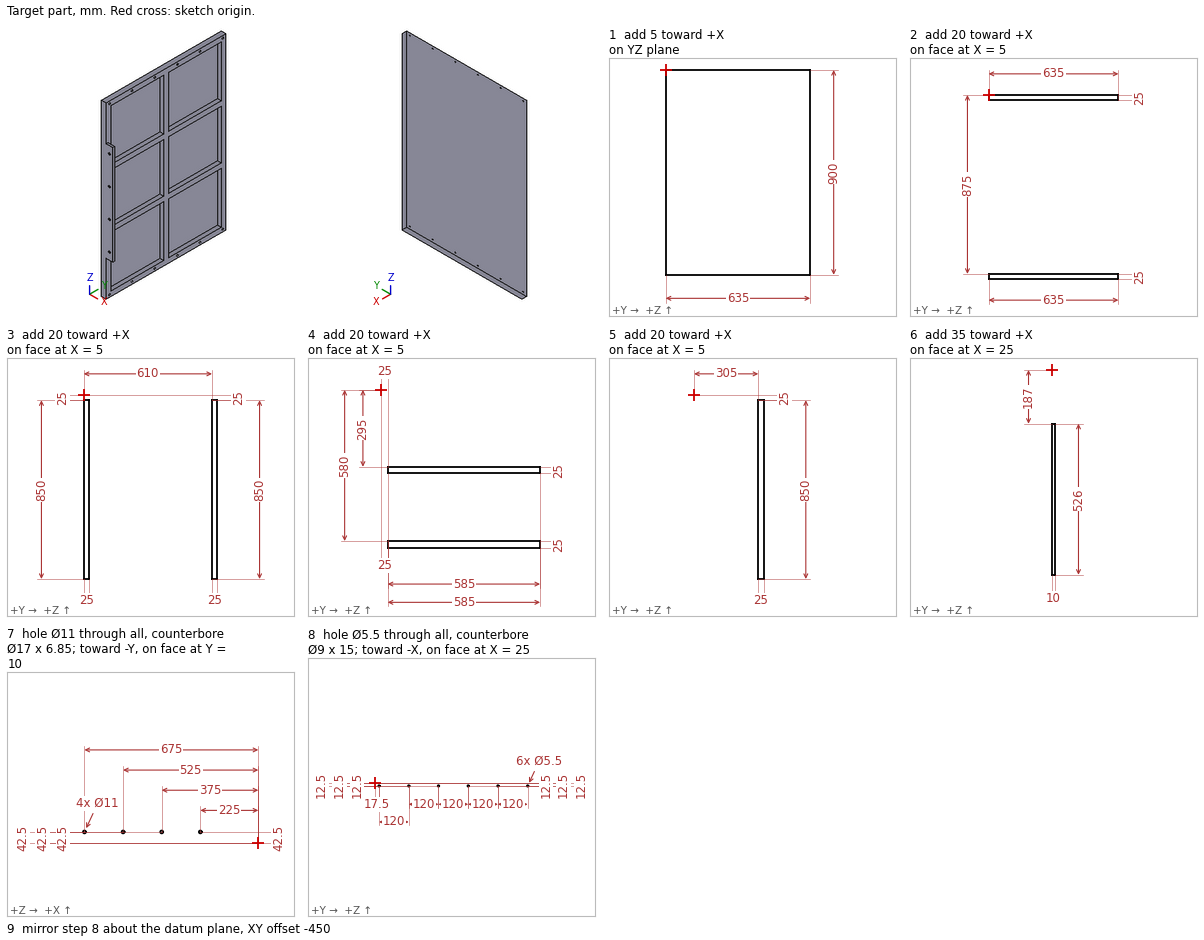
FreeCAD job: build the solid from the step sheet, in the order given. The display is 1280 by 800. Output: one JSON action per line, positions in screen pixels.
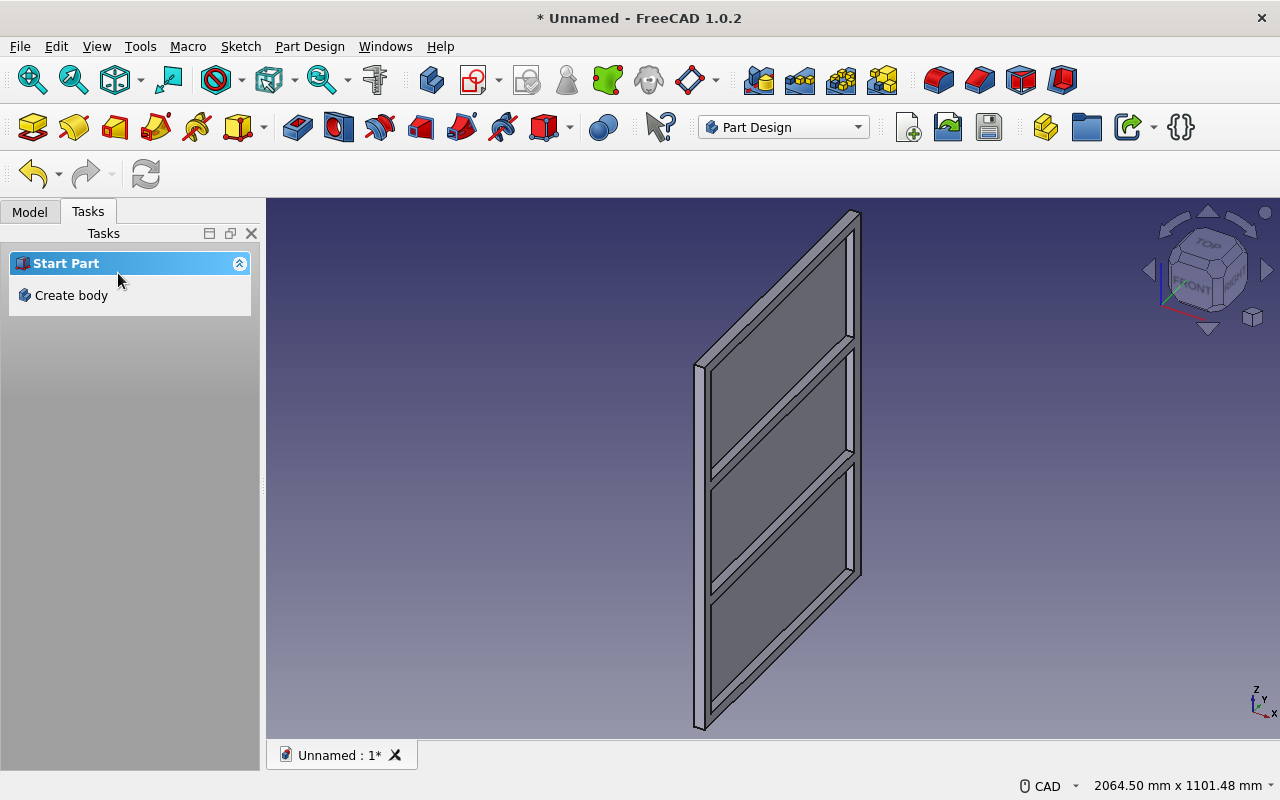
{"action": "left_click", "coordinate": [754, 372]}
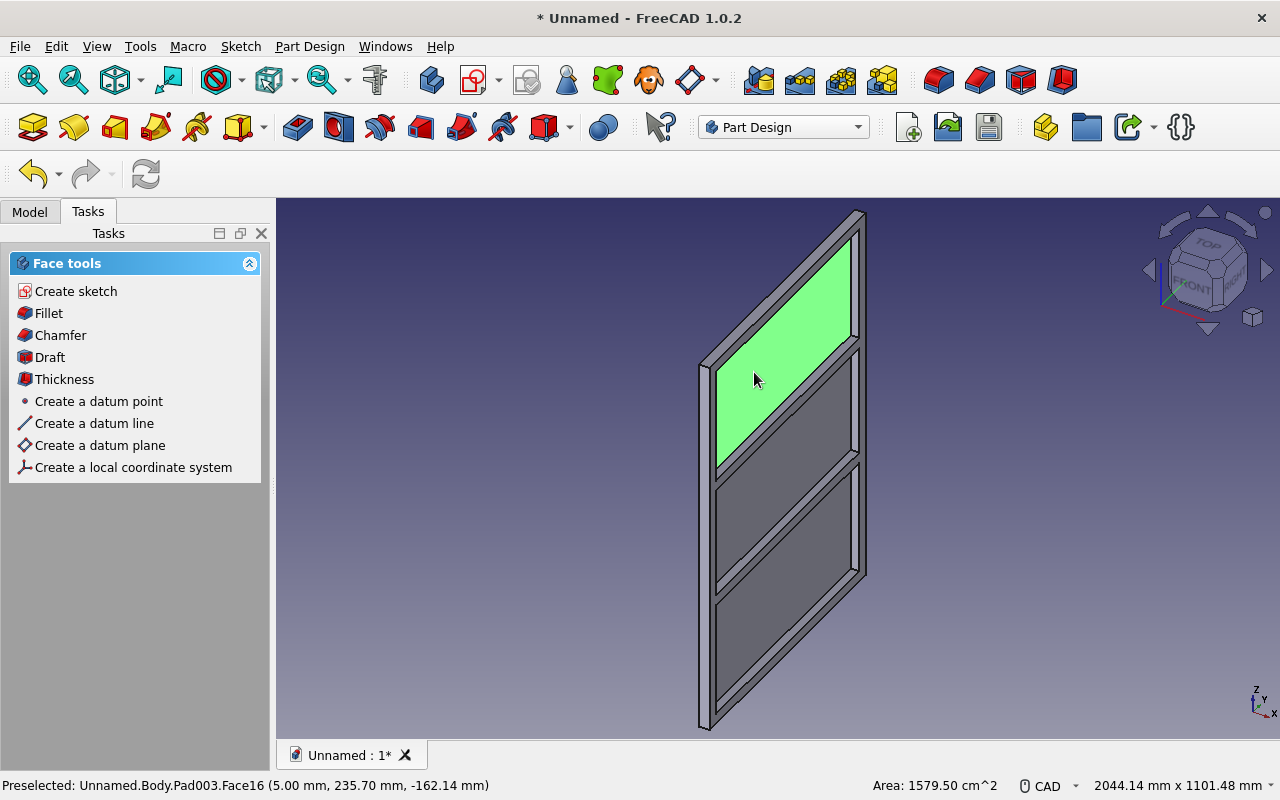
{"action": "left_click", "coordinate": [472, 80]}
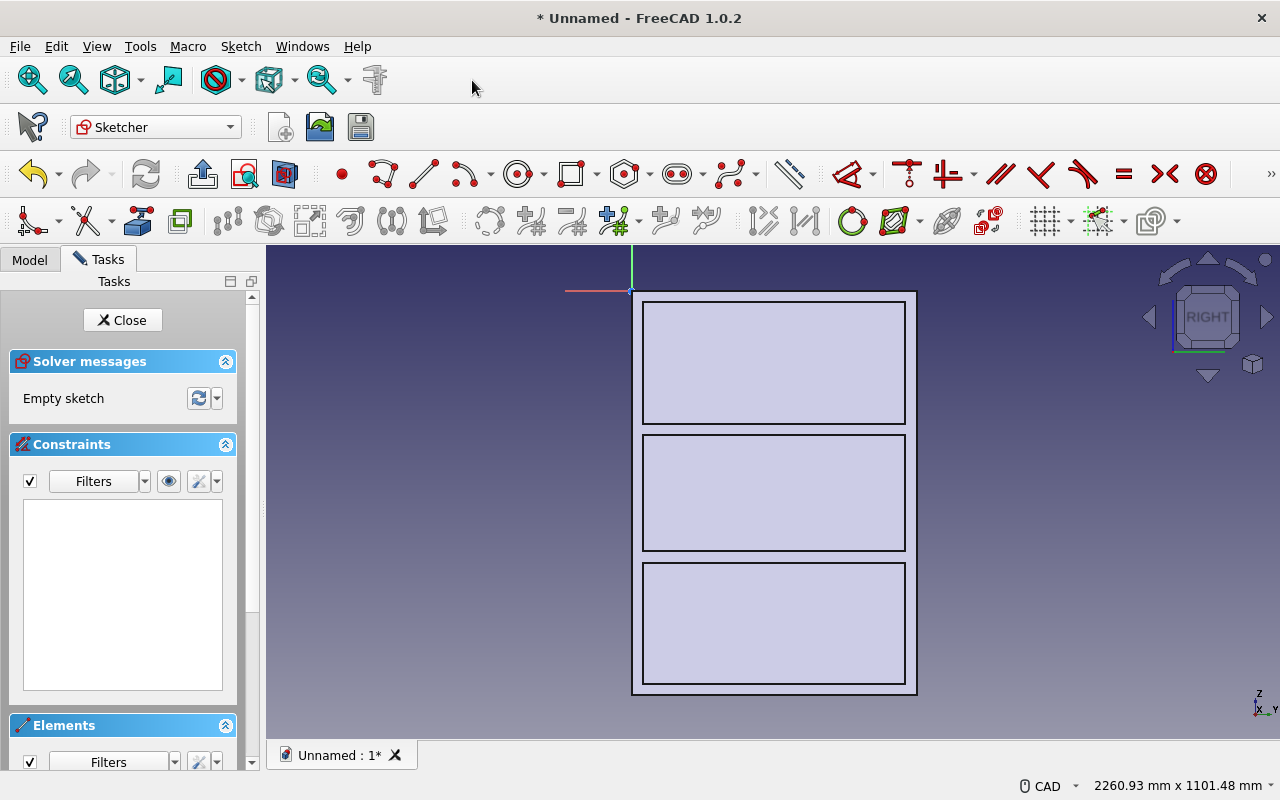
{"action": "scroll", "coordinate": [698, 513], "scroll_direction": "down", "scroll_amount": 1}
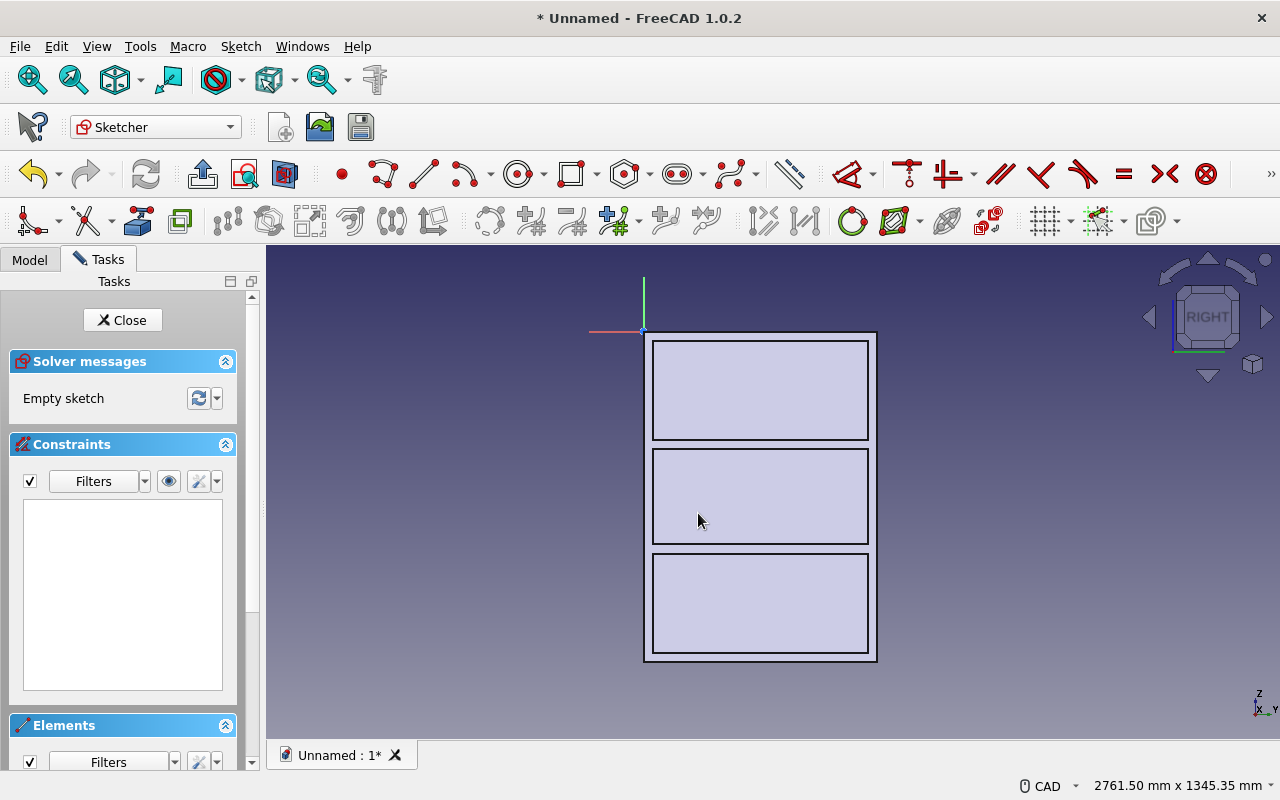
{"action": "left_click", "coordinate": [570, 174]}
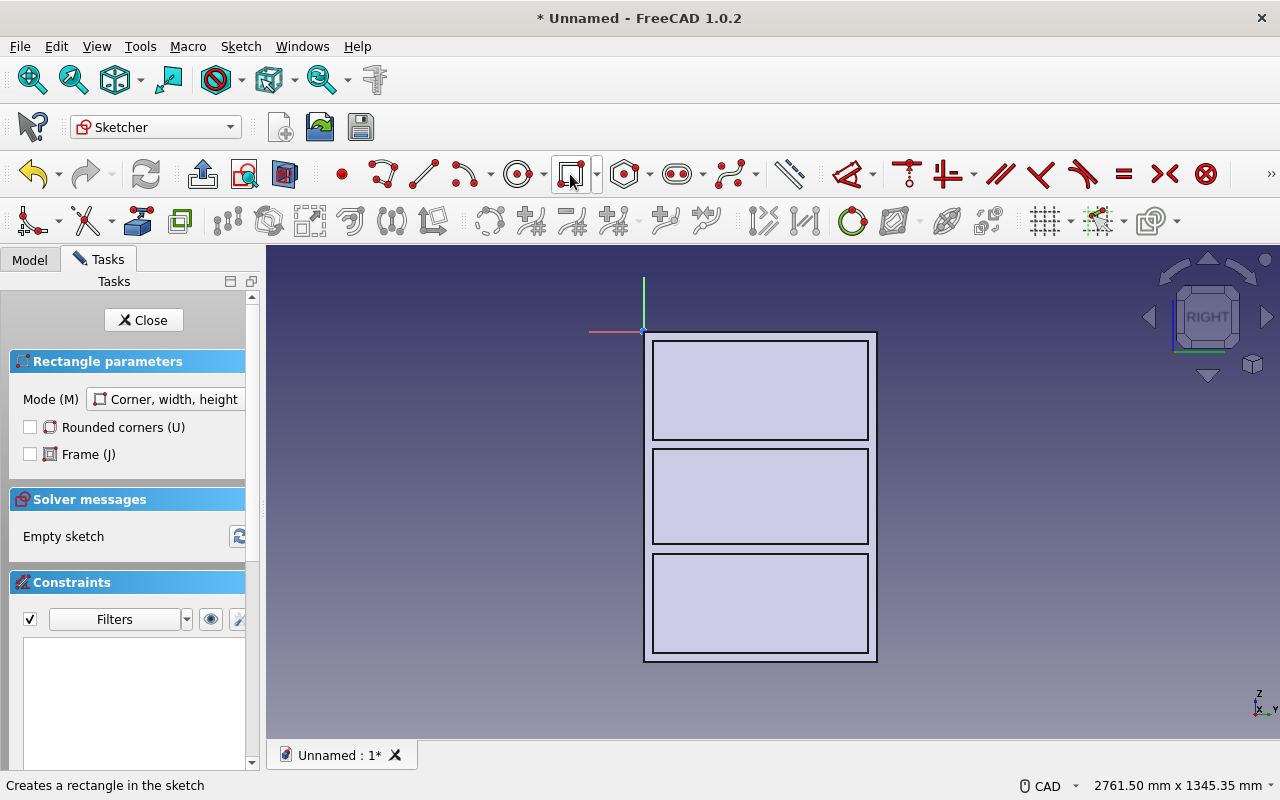
{"action": "scroll", "coordinate": [756, 341], "scroll_direction": "up", "scroll_amount": 3}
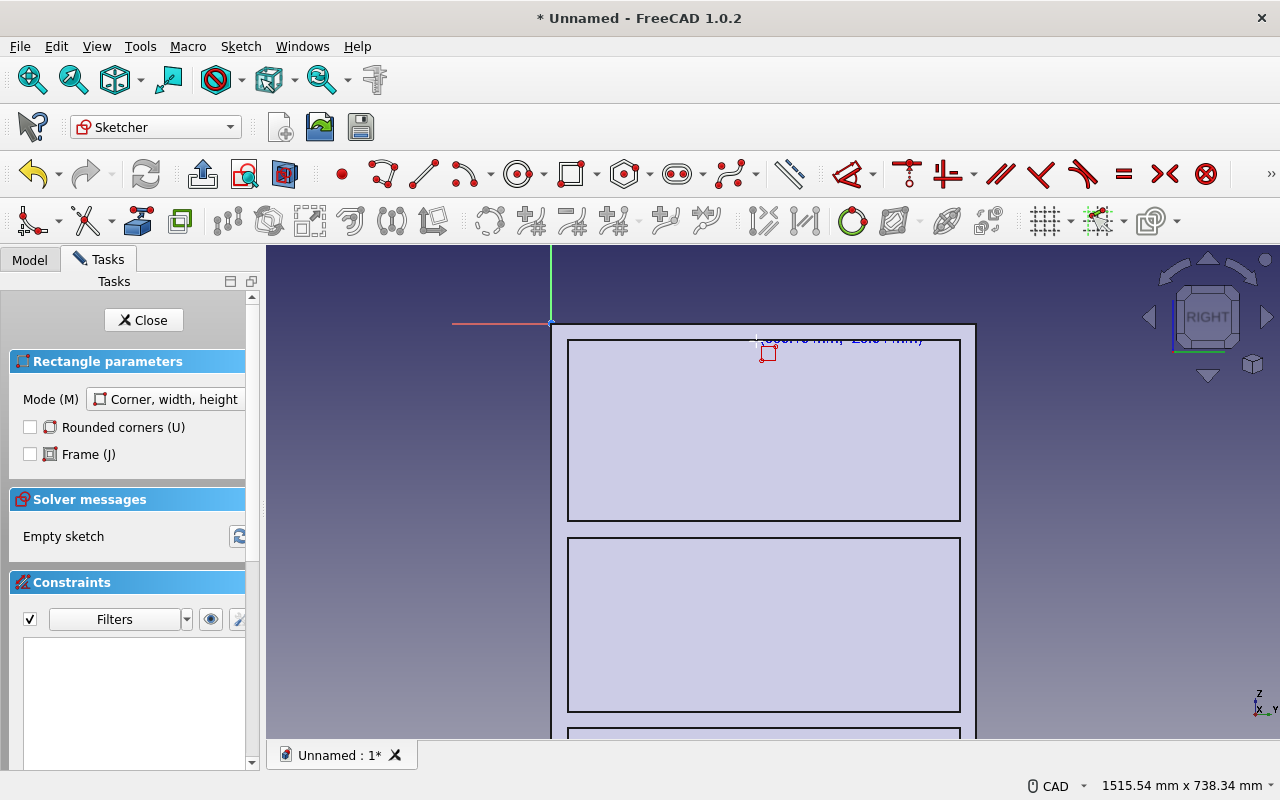
{"action": "left_click", "coordinate": [756, 340]}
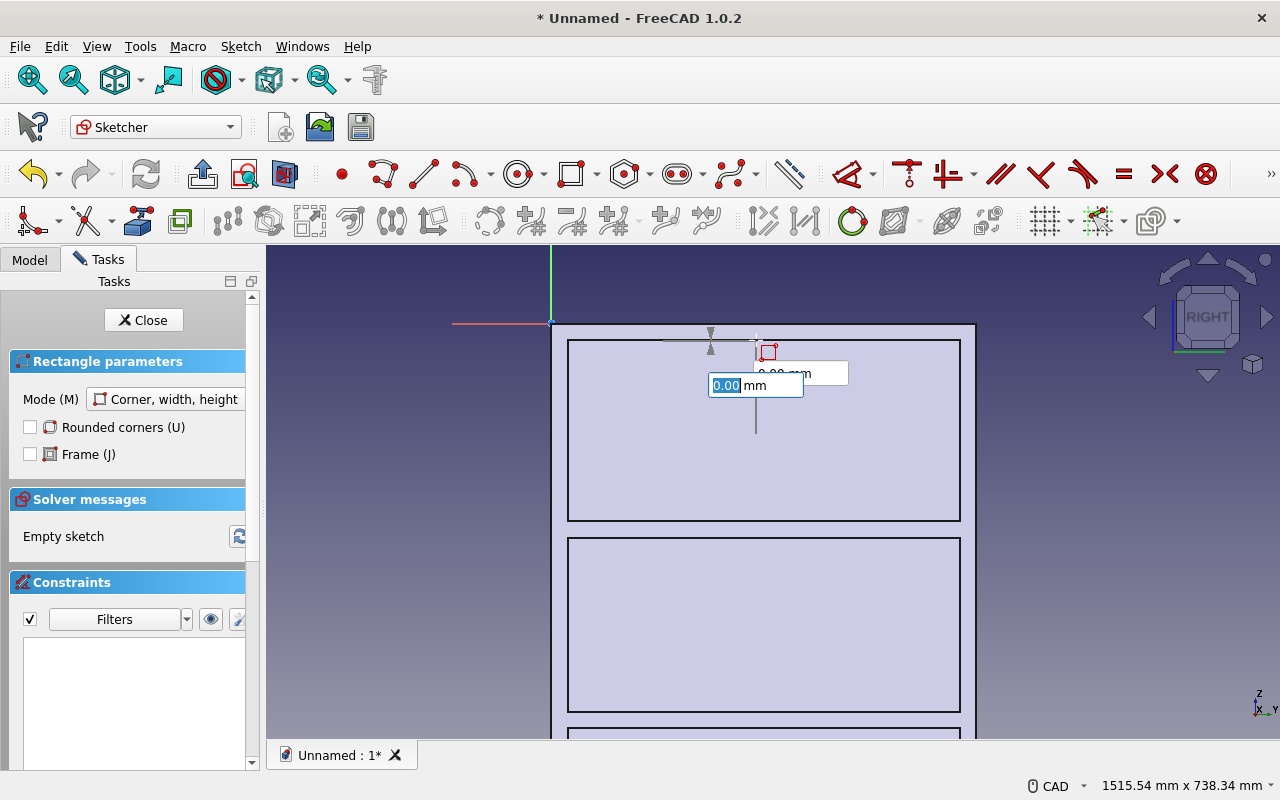
{"action": "scroll", "coordinate": [756, 341], "scroll_direction": "down", "scroll_amount": 3}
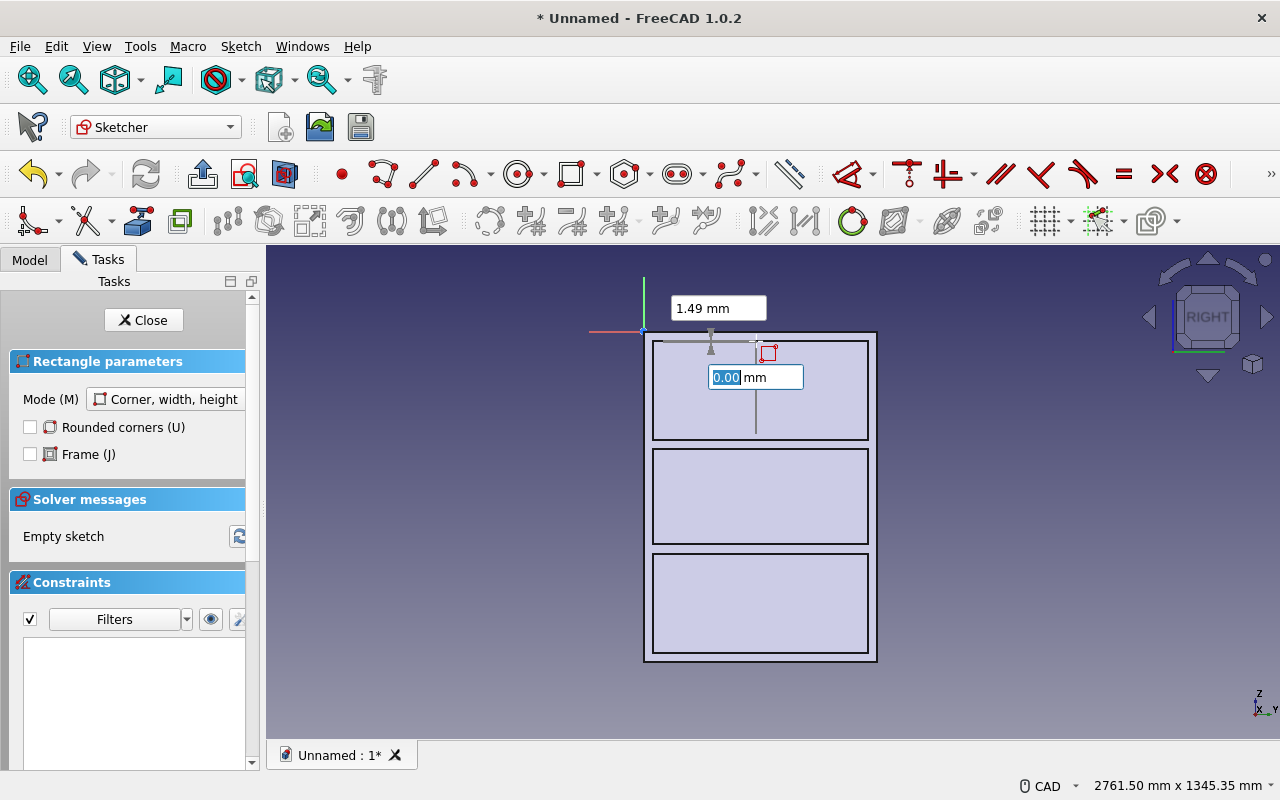
{"action": "left_click", "coordinate": [765, 653]}
{"action": "key", "text": "Escape"}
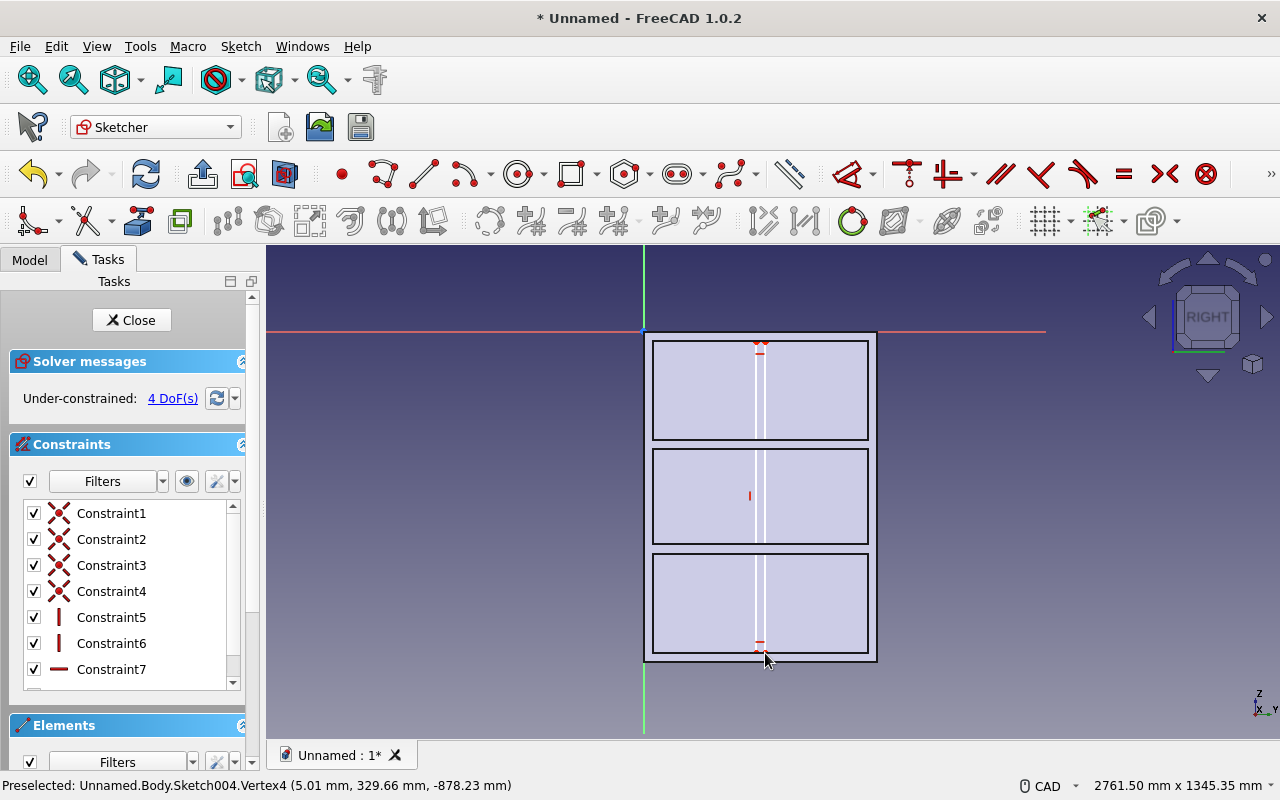
{"action": "key", "text": "d"}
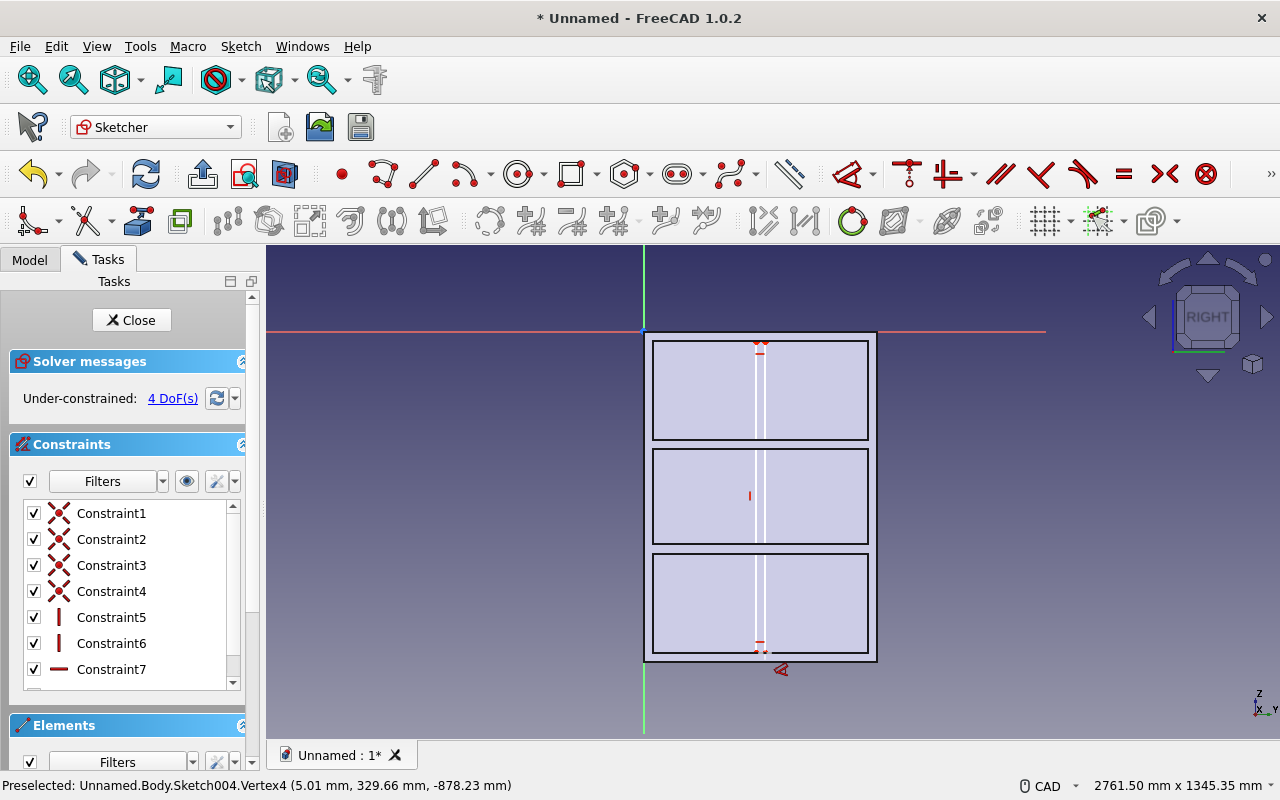
{"action": "scroll", "coordinate": [761, 654], "scroll_direction": "up", "scroll_amount": 8}